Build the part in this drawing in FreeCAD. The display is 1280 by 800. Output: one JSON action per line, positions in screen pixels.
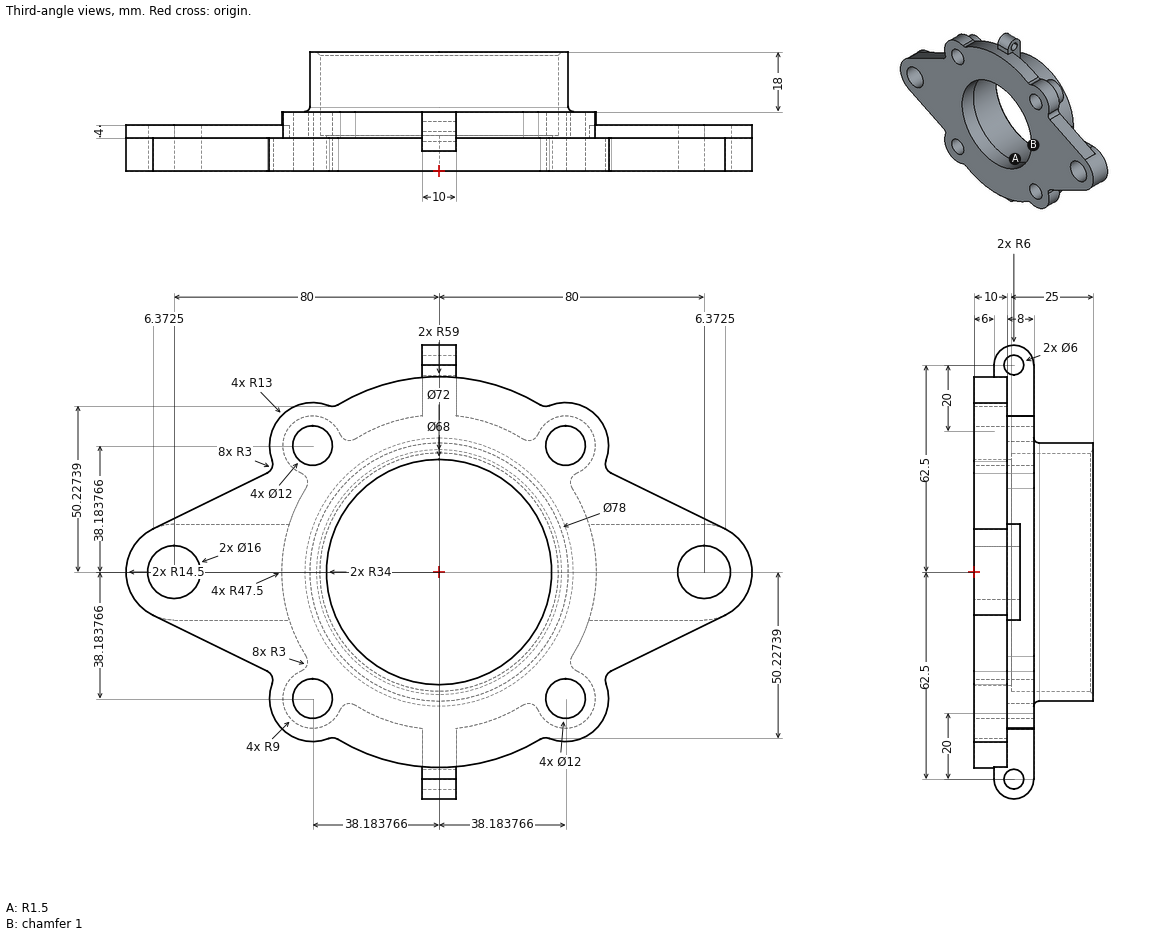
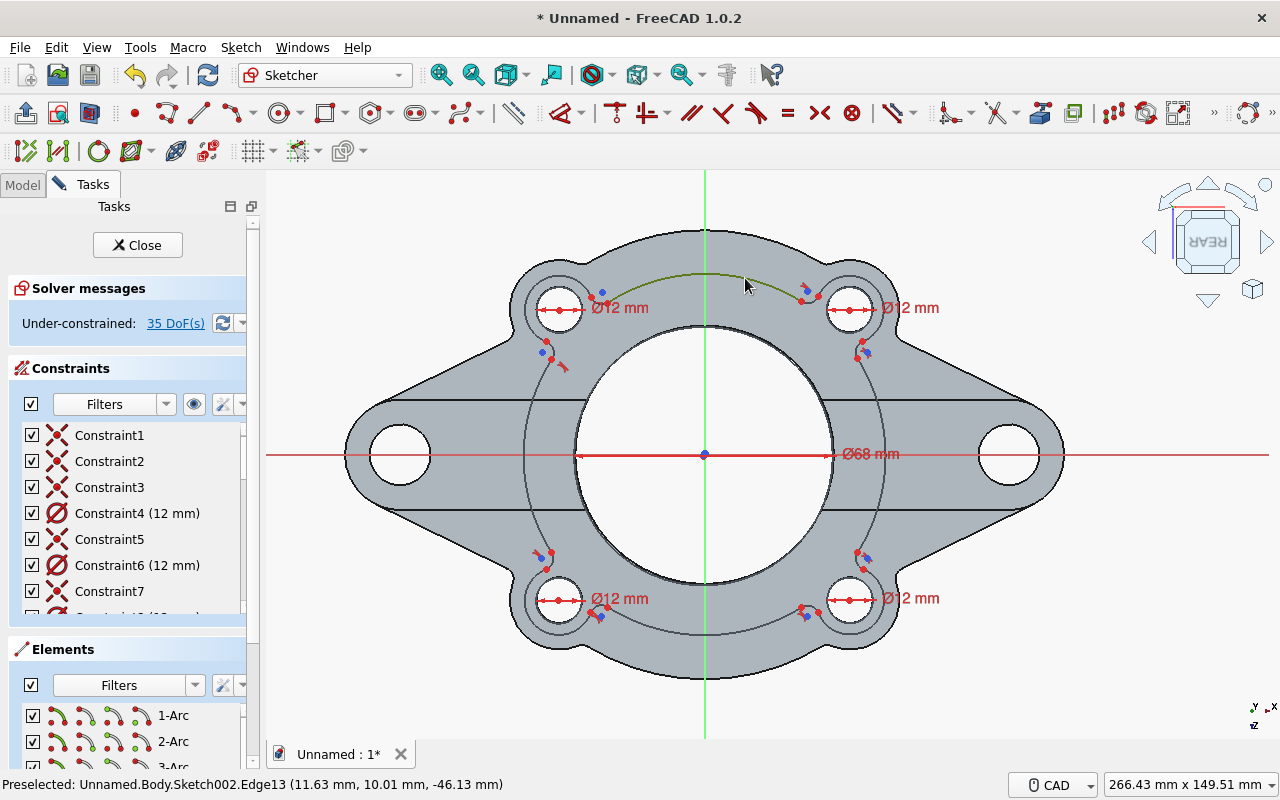
{"action": "scroll", "coordinate": [598, 304], "scroll_direction": "up", "scroll_amount": 3}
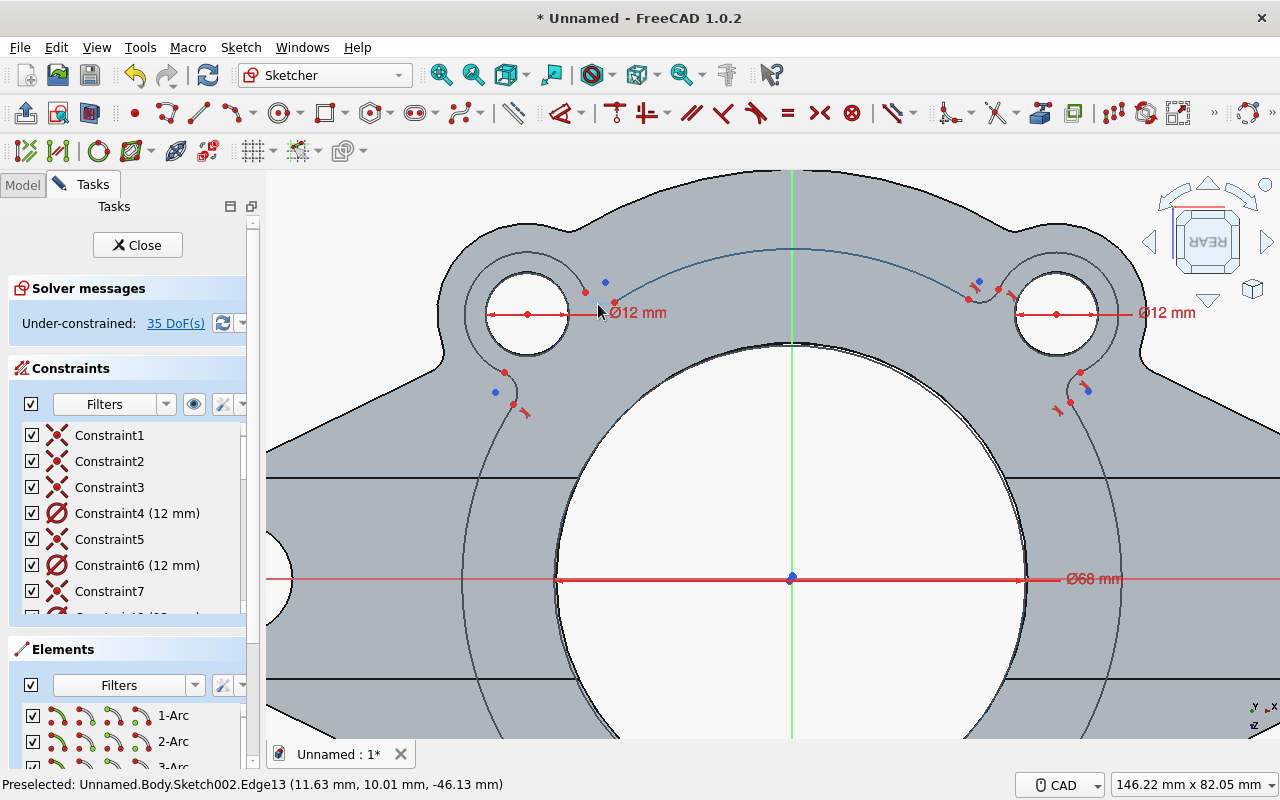
{"action": "left_click", "coordinate": [598, 303]}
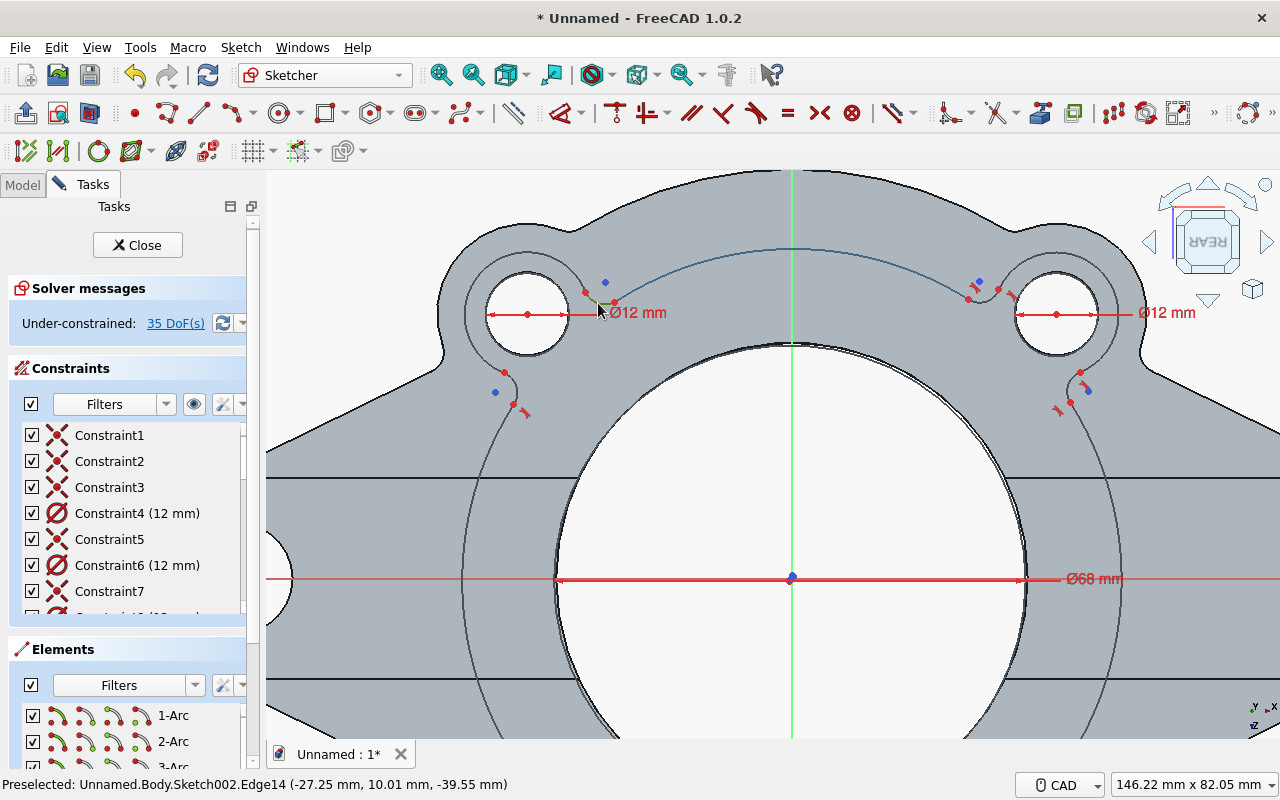
{"action": "left_click", "coordinate": [756, 114]}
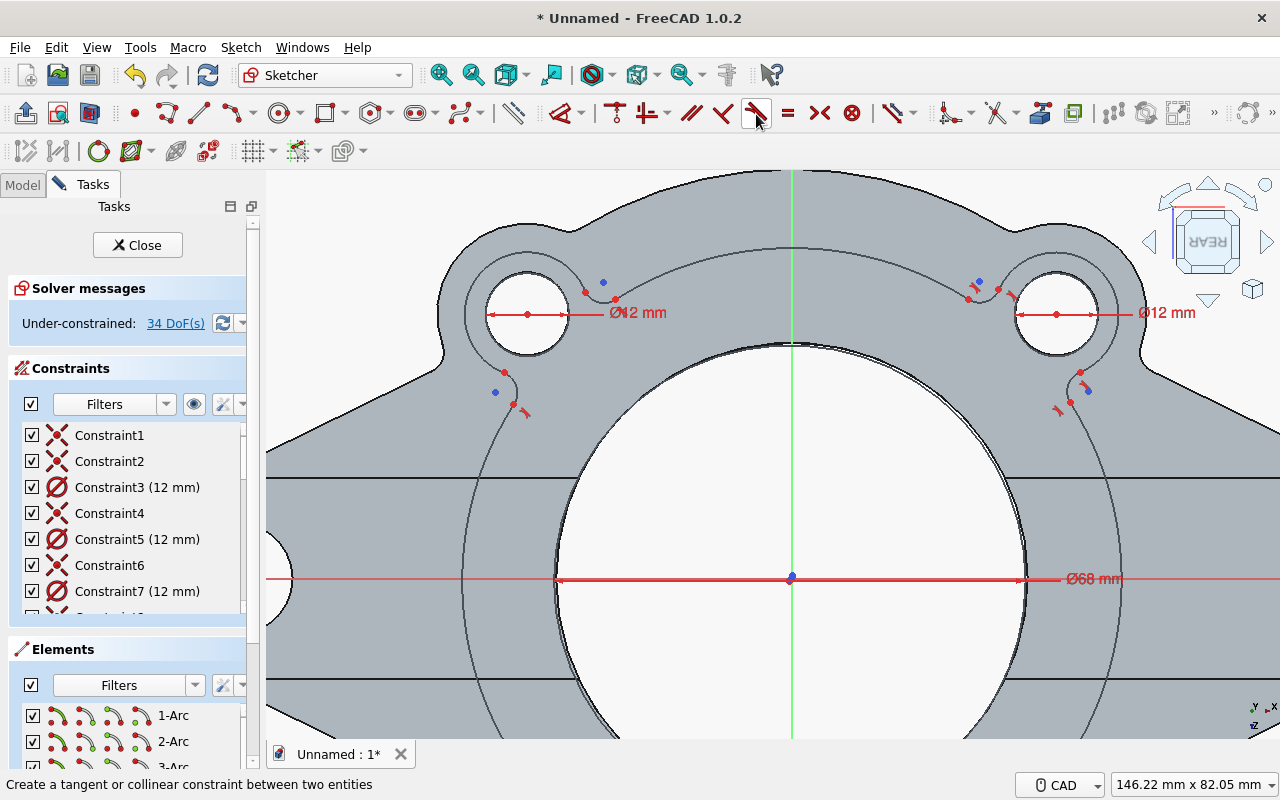
{"action": "scroll", "coordinate": [592, 300], "scroll_direction": "up", "scroll_amount": 2}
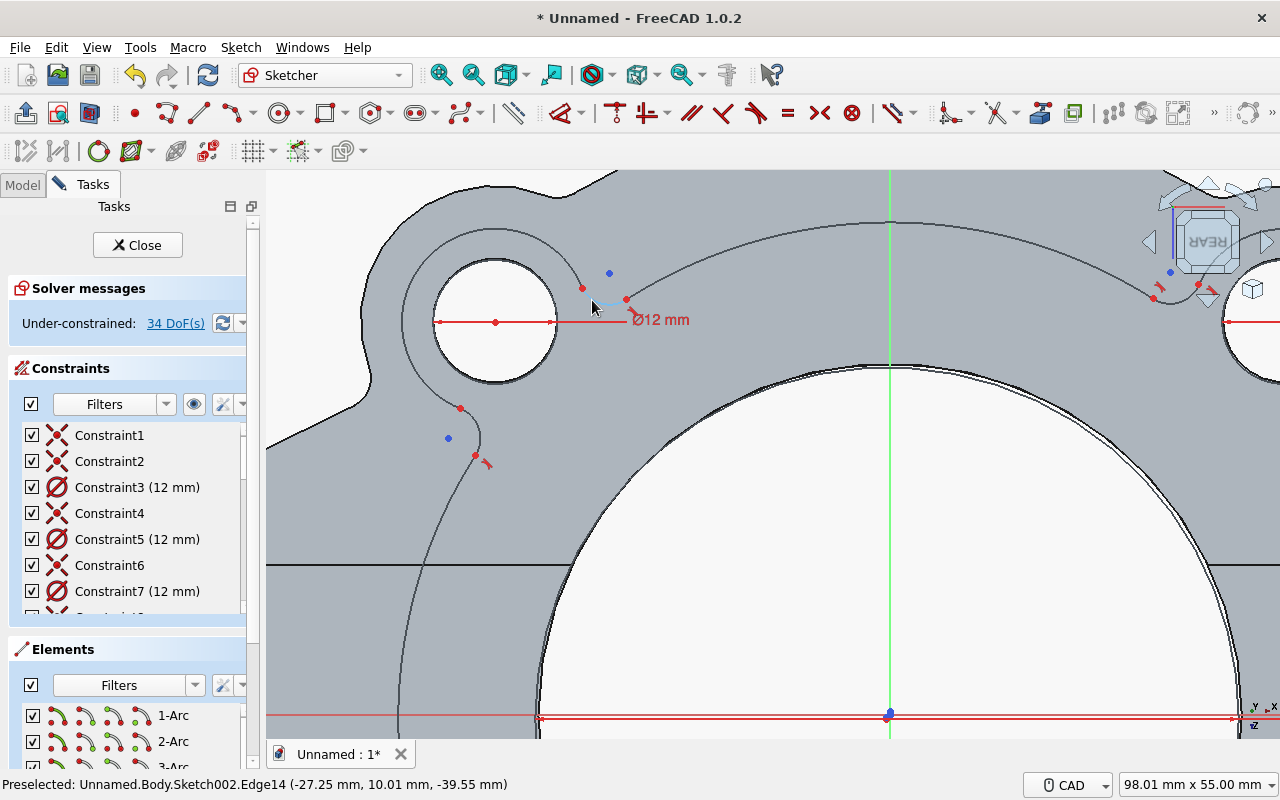
{"action": "left_click", "coordinate": [593, 300]}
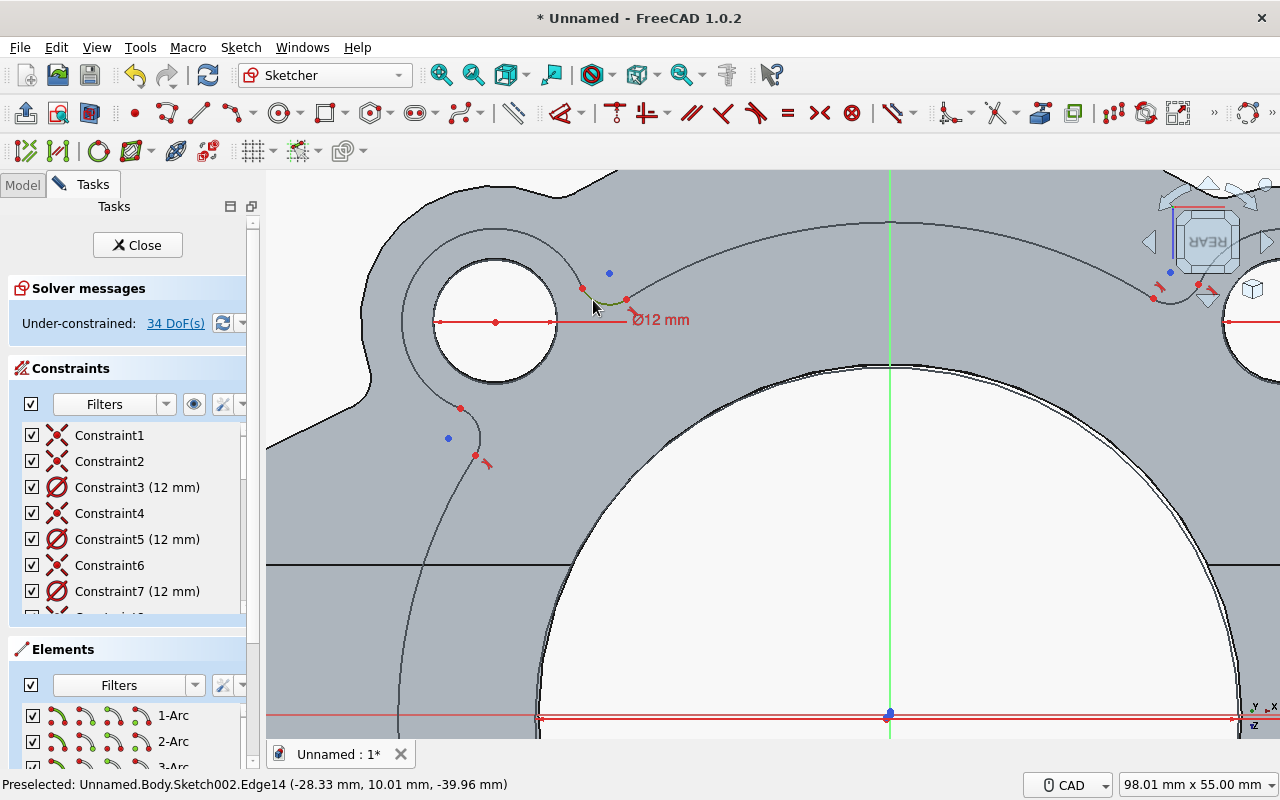
{"action": "left_click", "coordinate": [497, 229]}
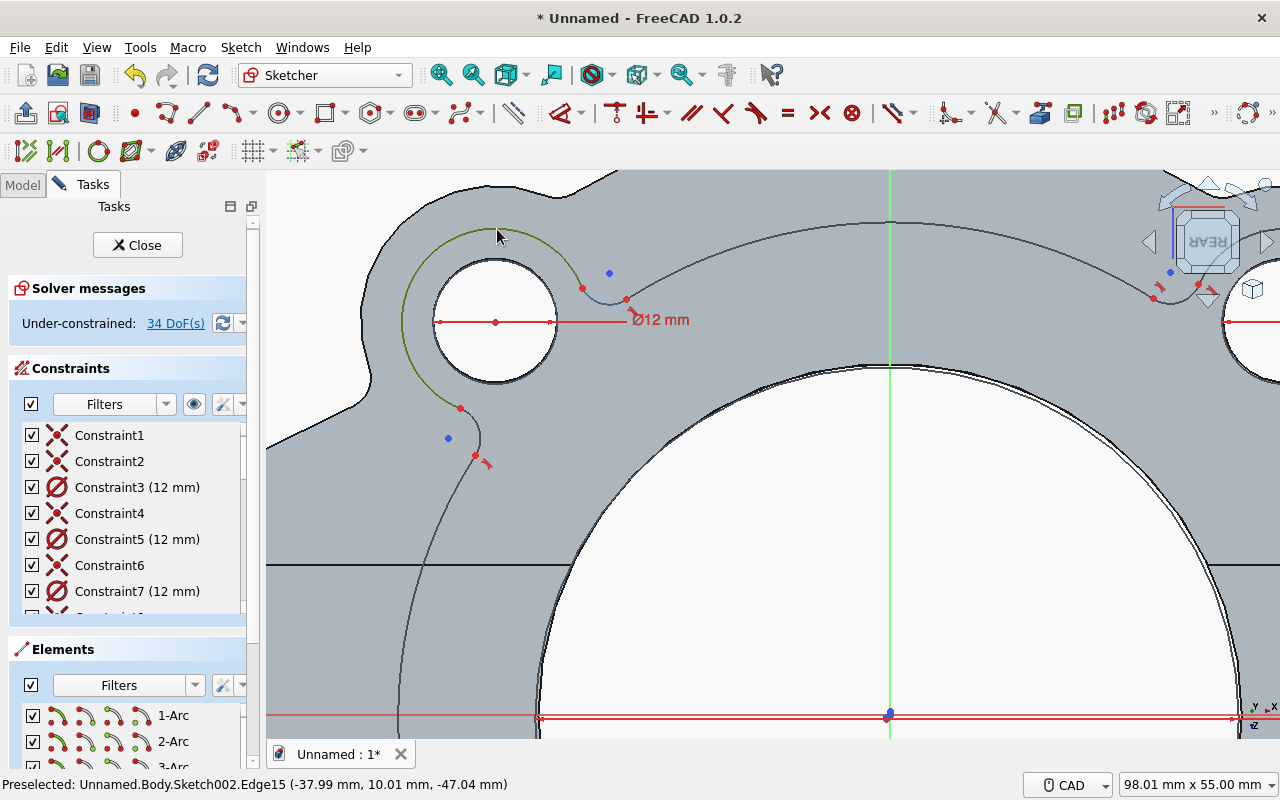
{"action": "left_click", "coordinate": [756, 114]}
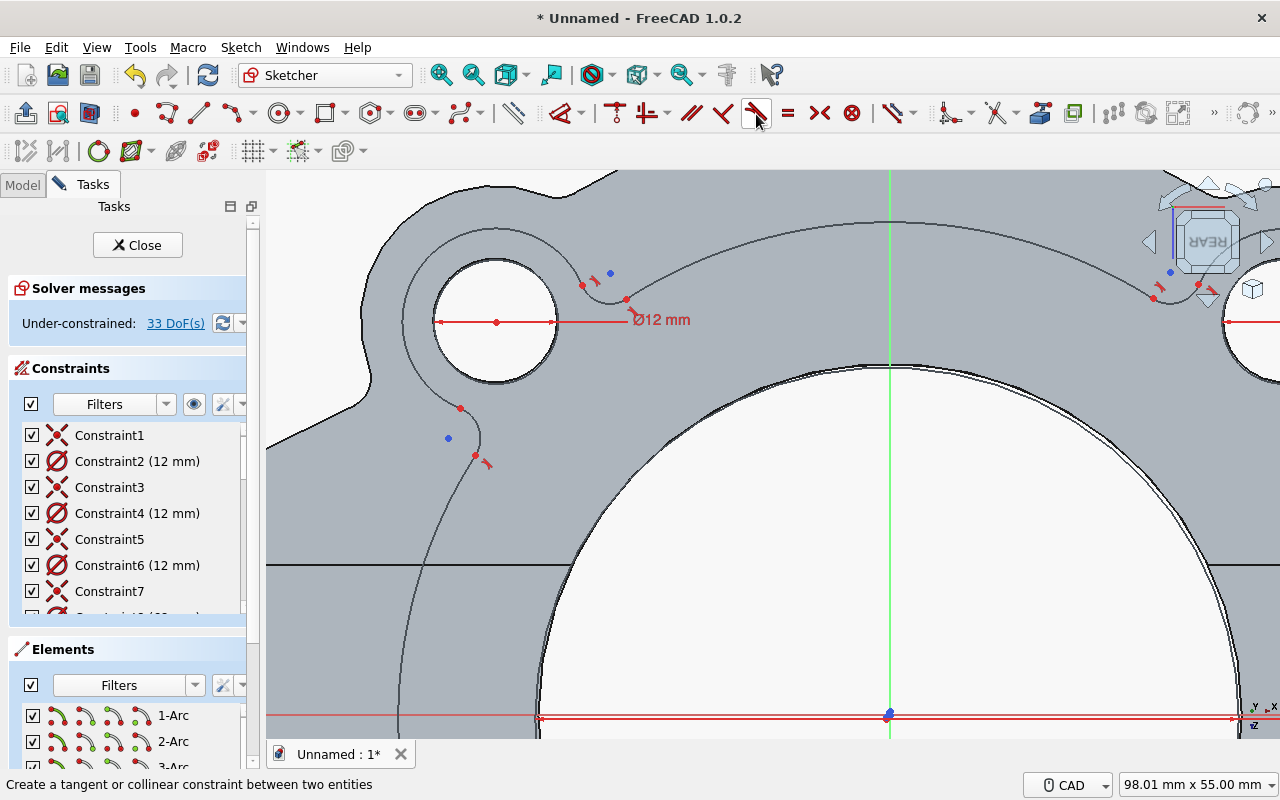
{"action": "left_click", "coordinate": [495, 228]}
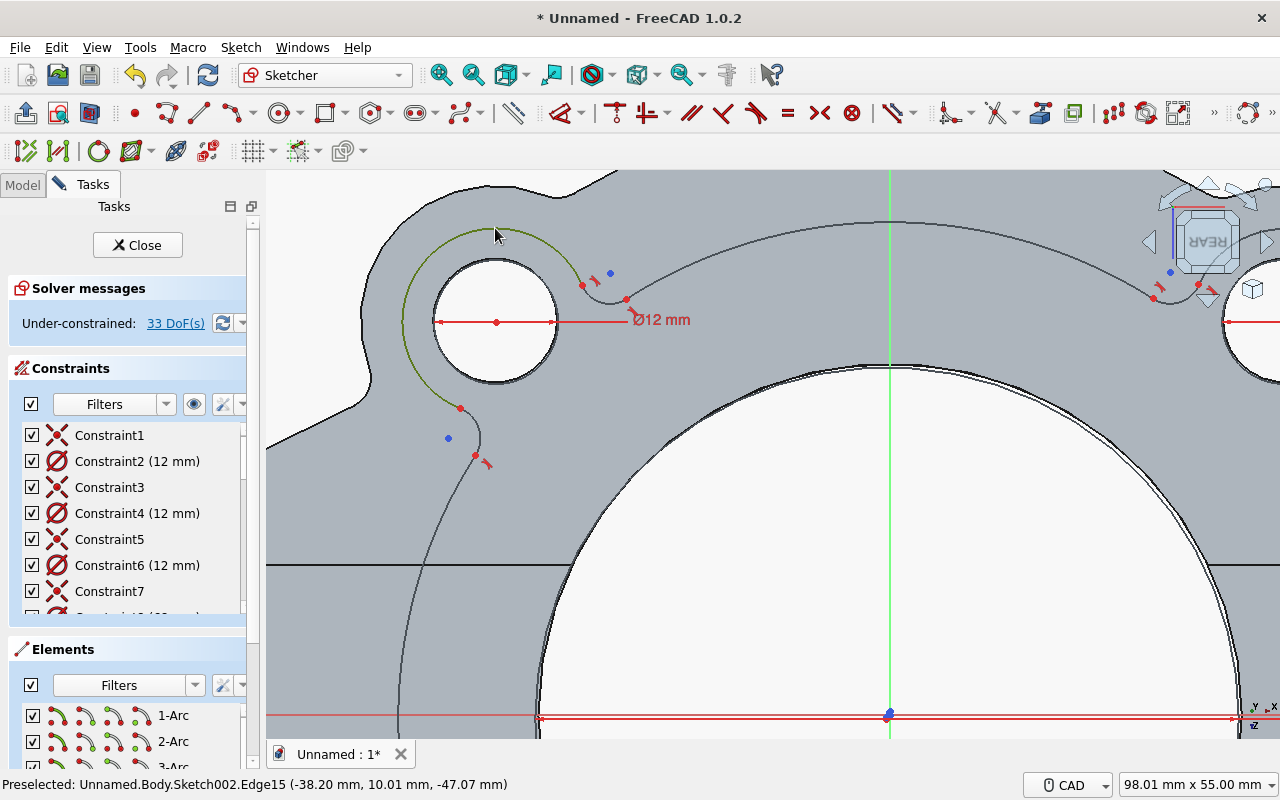
{"action": "left_click", "coordinate": [480, 440]}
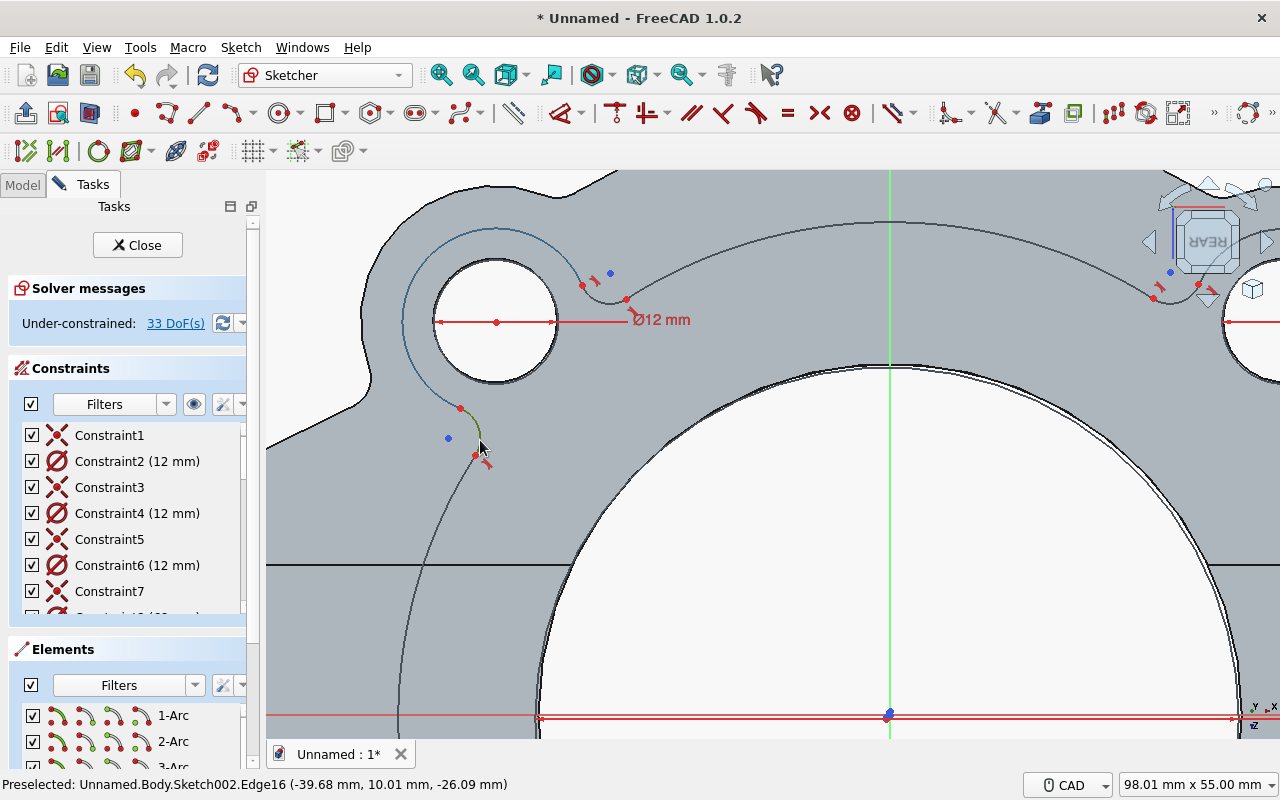
{"action": "left_click", "coordinate": [756, 114]}